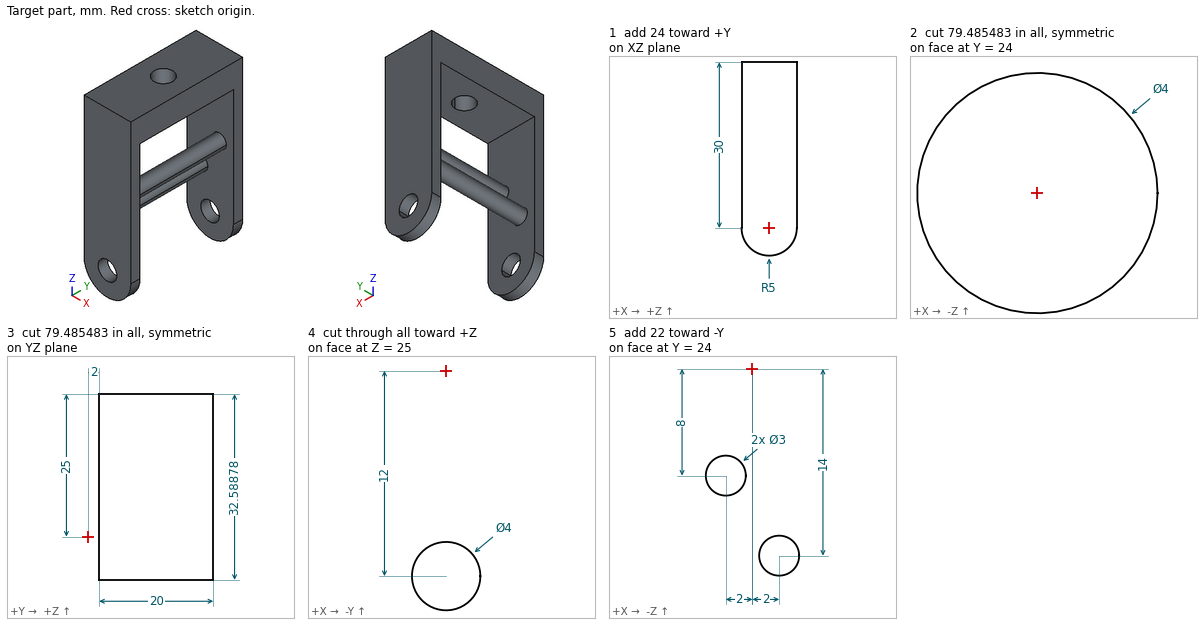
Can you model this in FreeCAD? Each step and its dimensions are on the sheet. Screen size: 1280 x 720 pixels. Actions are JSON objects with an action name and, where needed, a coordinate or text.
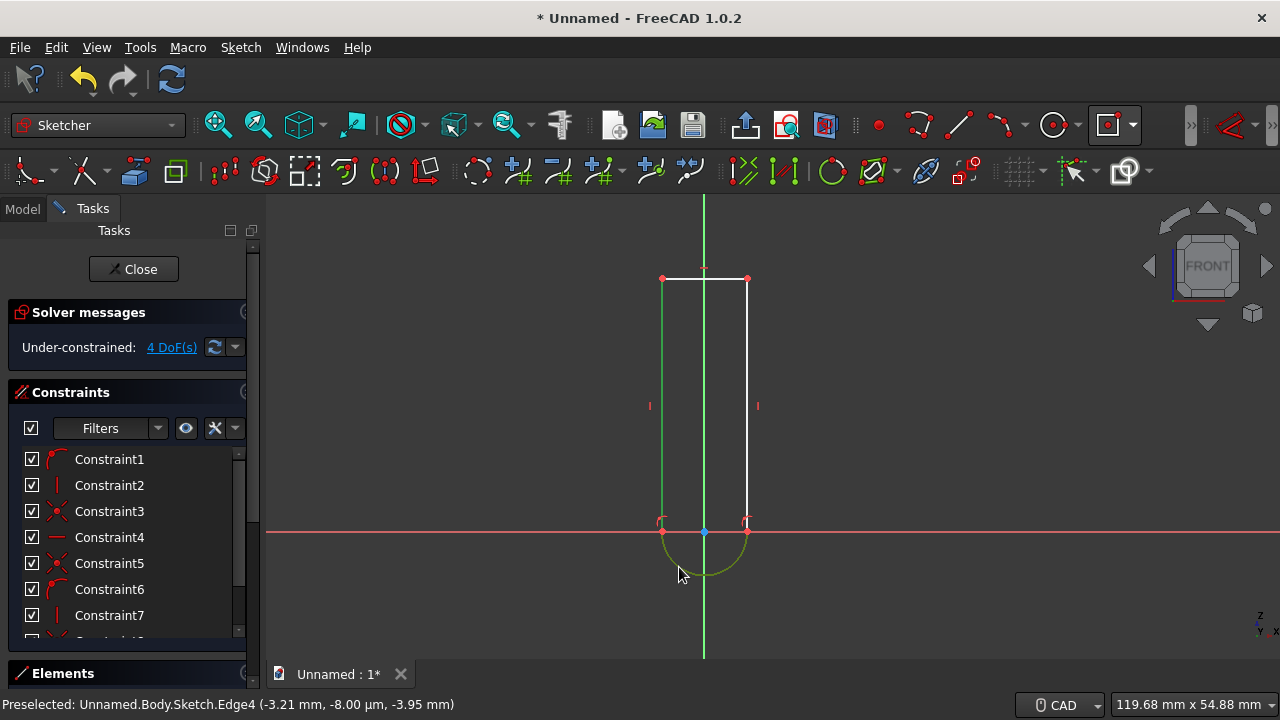
{"action": "key", "text": "t"}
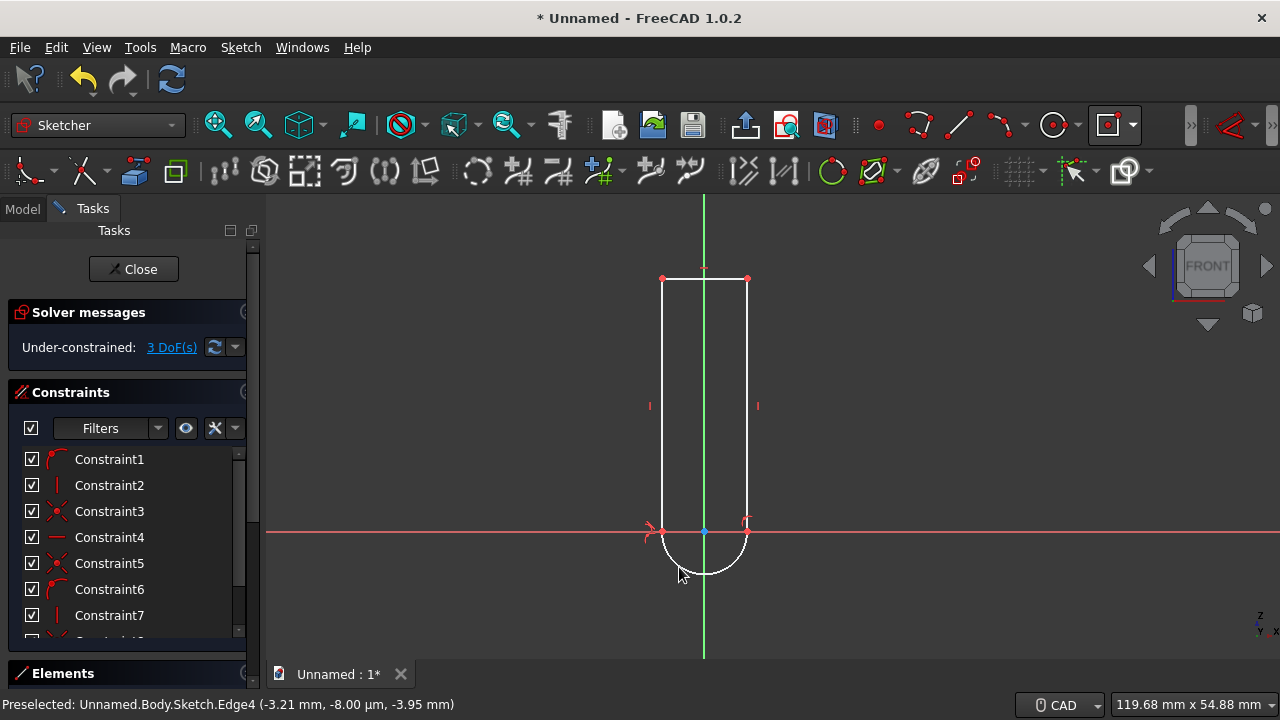
{"action": "left_click", "coordinate": [704, 532]}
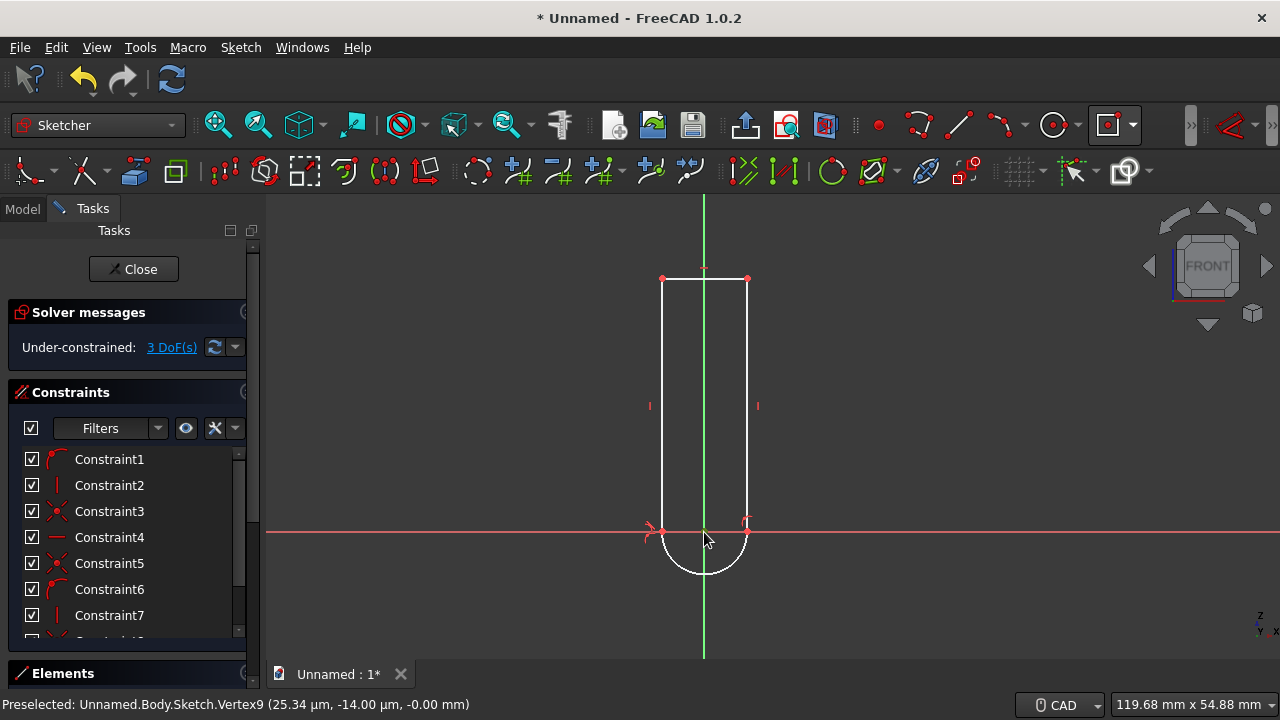
{"action": "left_click", "coordinate": [704, 485]}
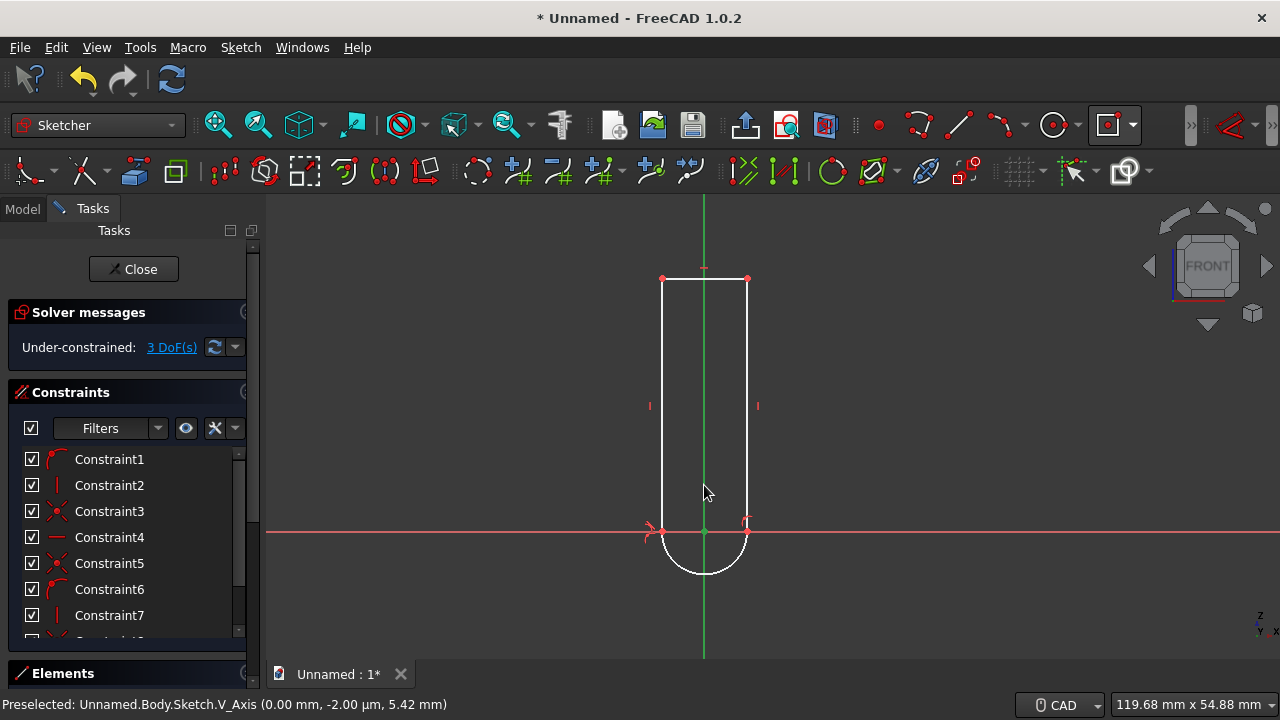
{"action": "key", "text": "c"}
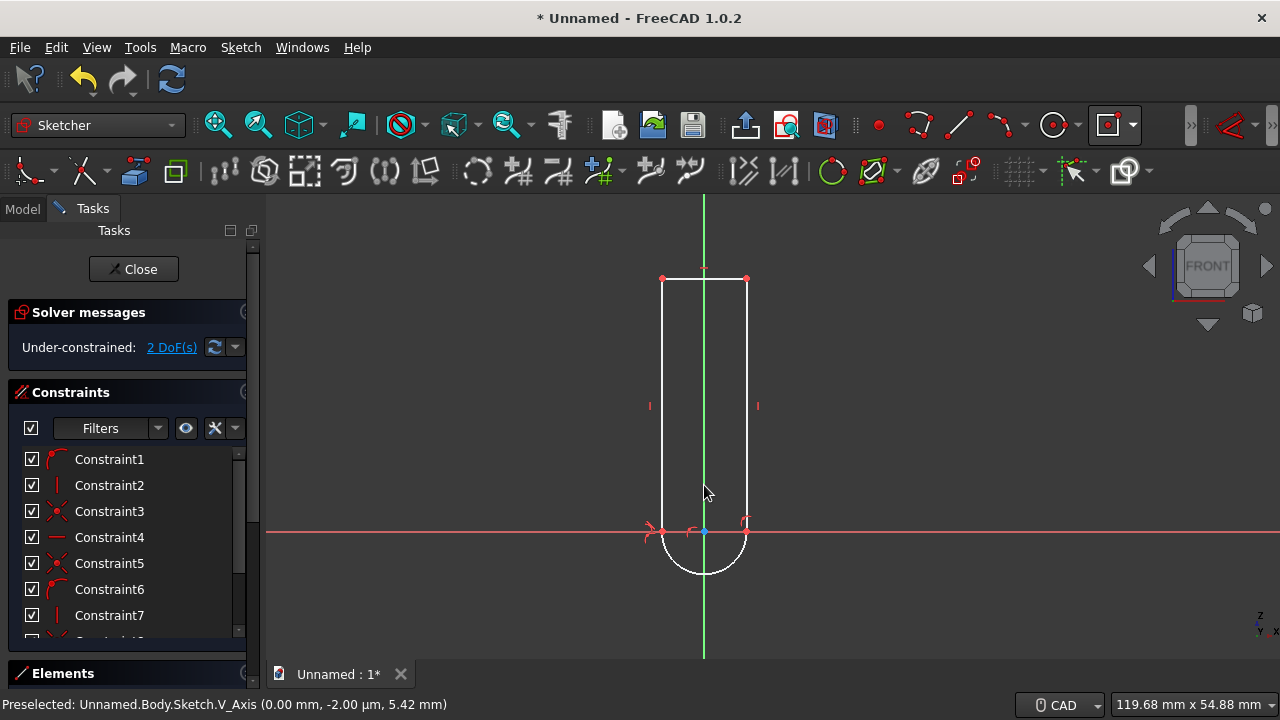
{"action": "left_click", "coordinate": [1230, 126]}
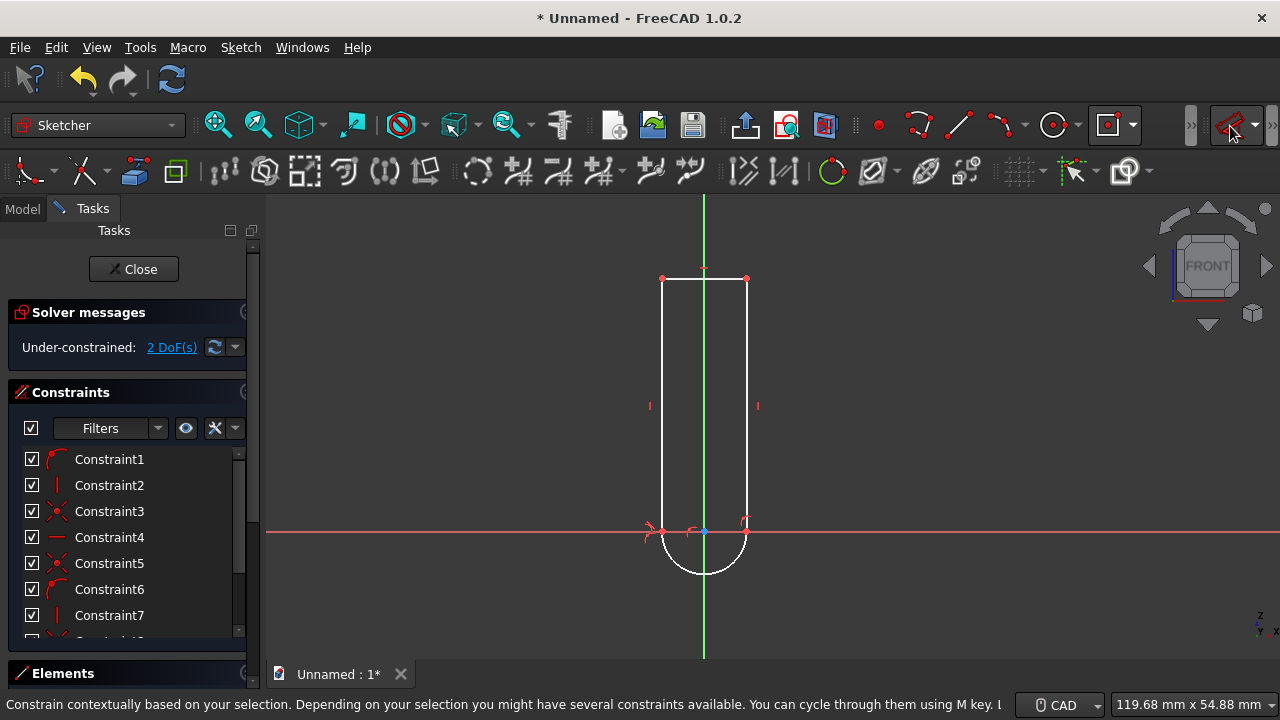
{"action": "left_click", "coordinate": [679, 566]}
{"action": "left_click", "coordinate": [660, 592]}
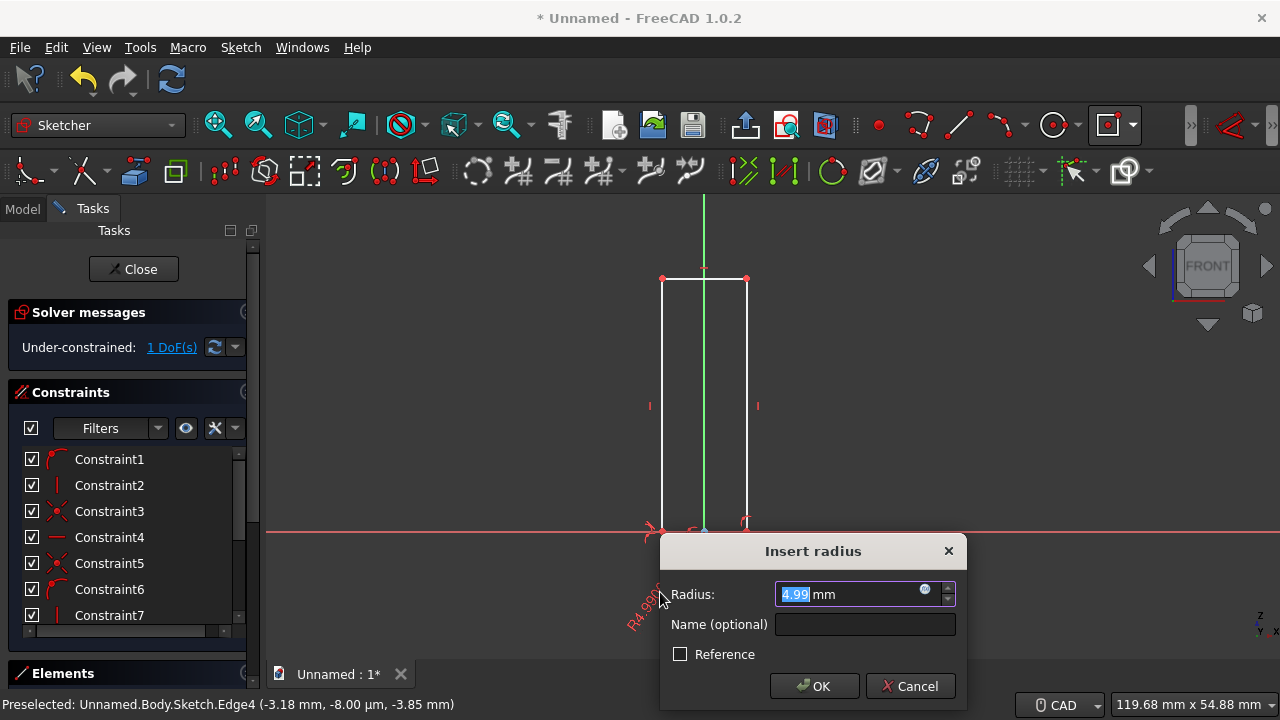
{"action": "type", "text": "5"}
{"action": "key", "text": "Return"}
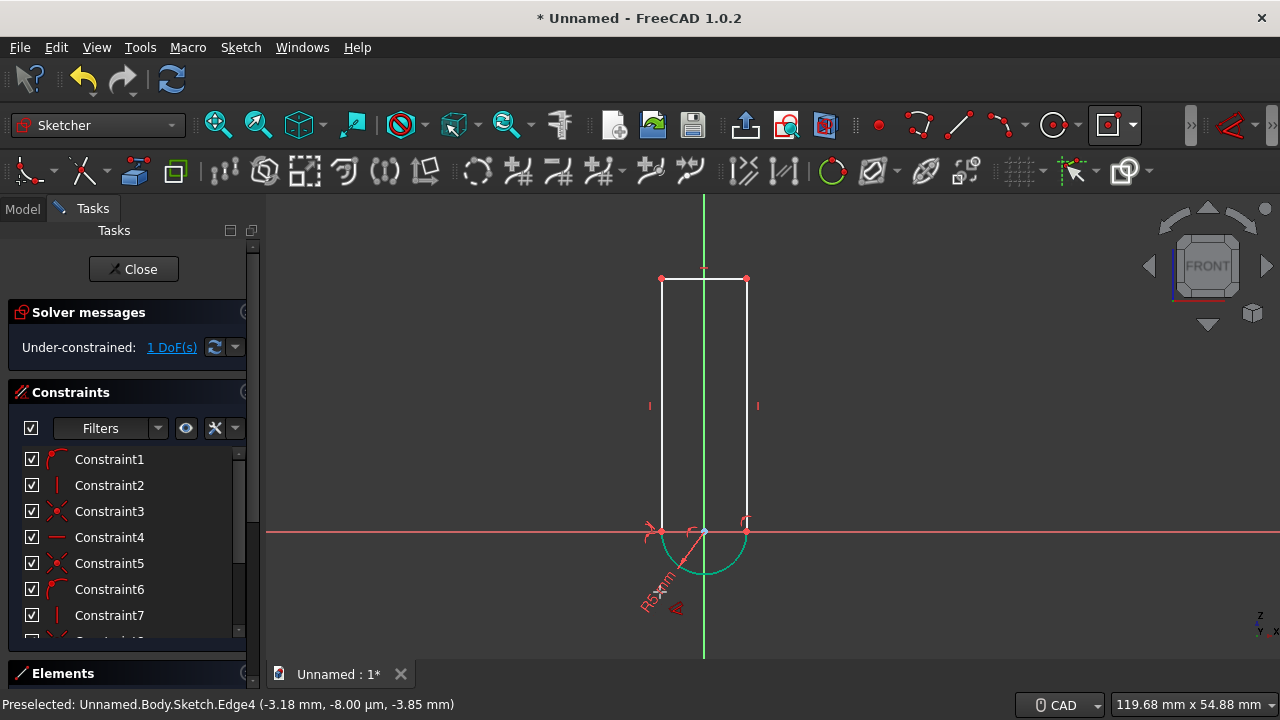
{"action": "left_click", "coordinate": [662, 456]}
{"action": "left_click", "coordinate": [628, 405]}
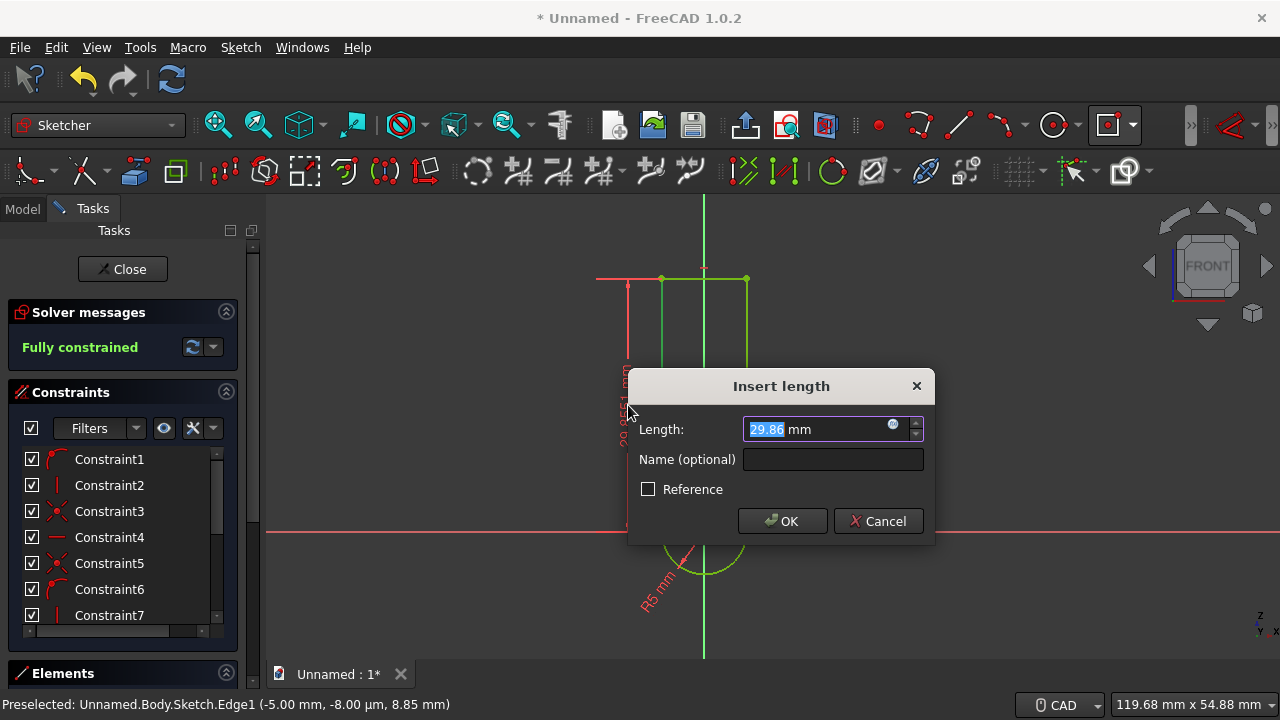
{"action": "type", "text": "30"}
{"action": "key", "text": "Return"}
{"action": "key", "text": "Escape"}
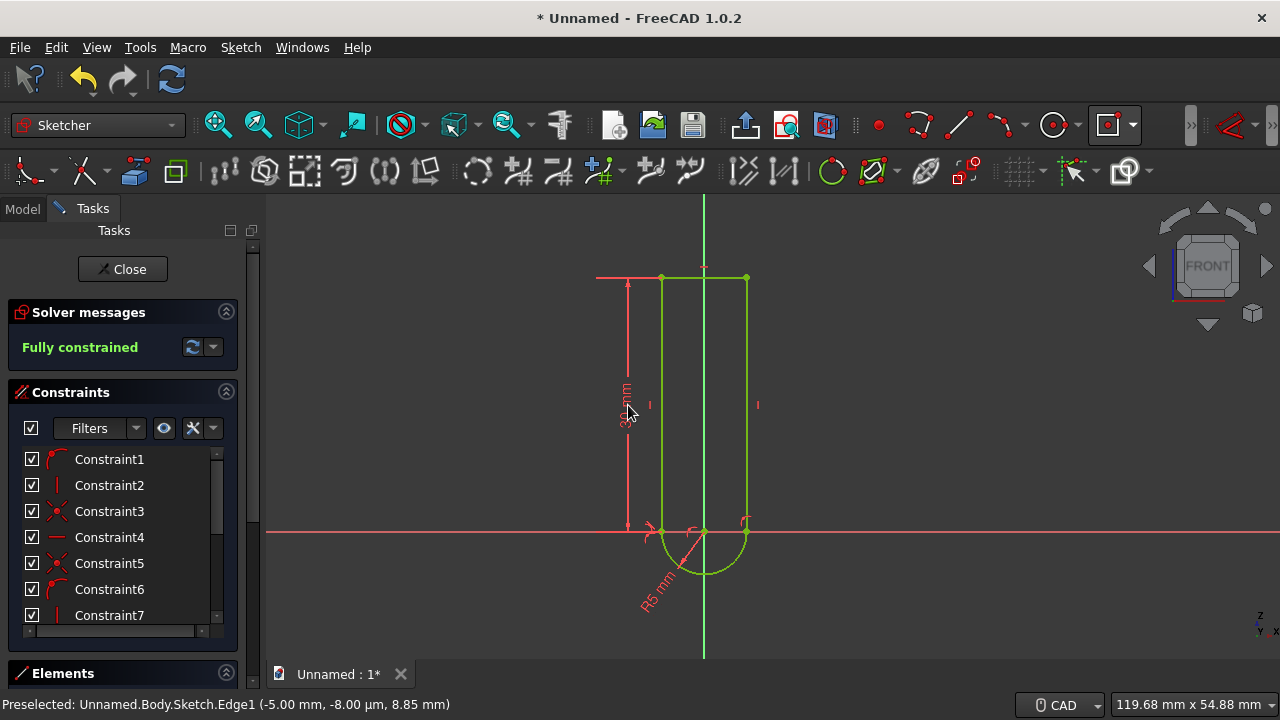
{"action": "left_click", "coordinate": [123, 269]}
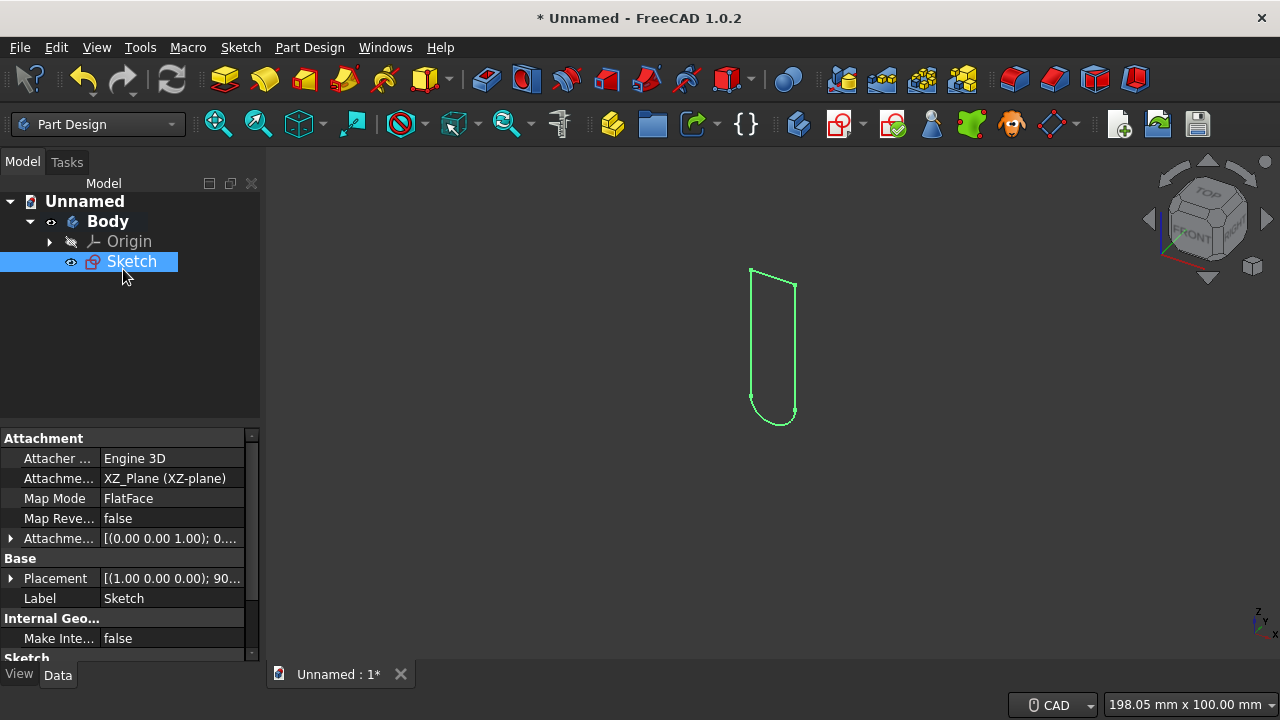
{"action": "left_click", "coordinate": [226, 80]}